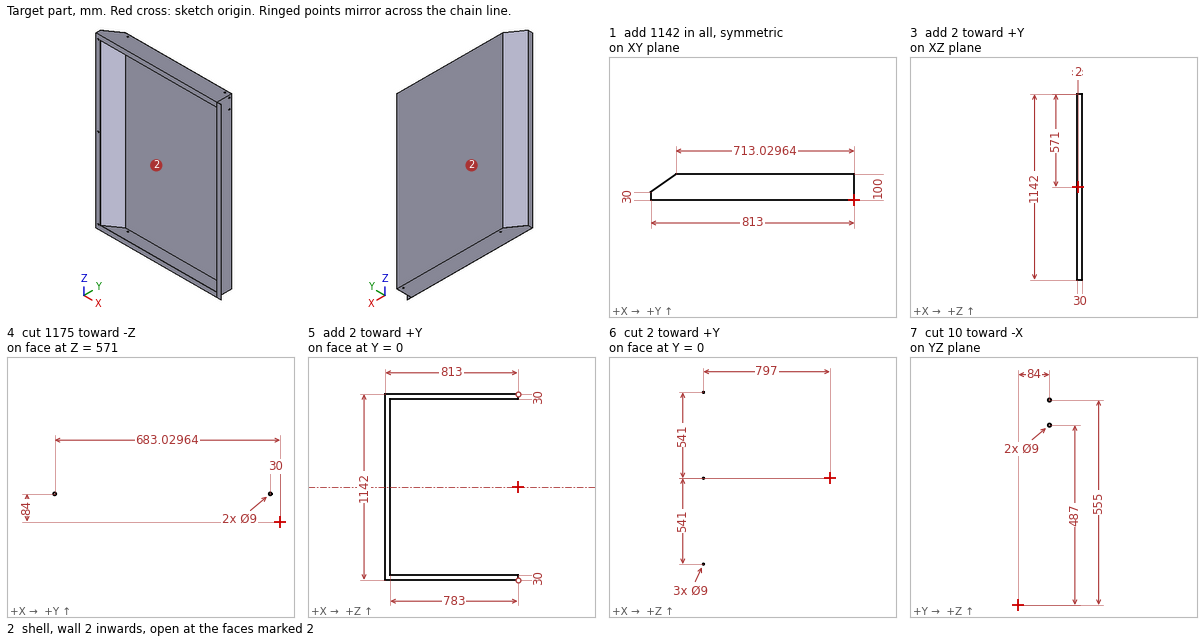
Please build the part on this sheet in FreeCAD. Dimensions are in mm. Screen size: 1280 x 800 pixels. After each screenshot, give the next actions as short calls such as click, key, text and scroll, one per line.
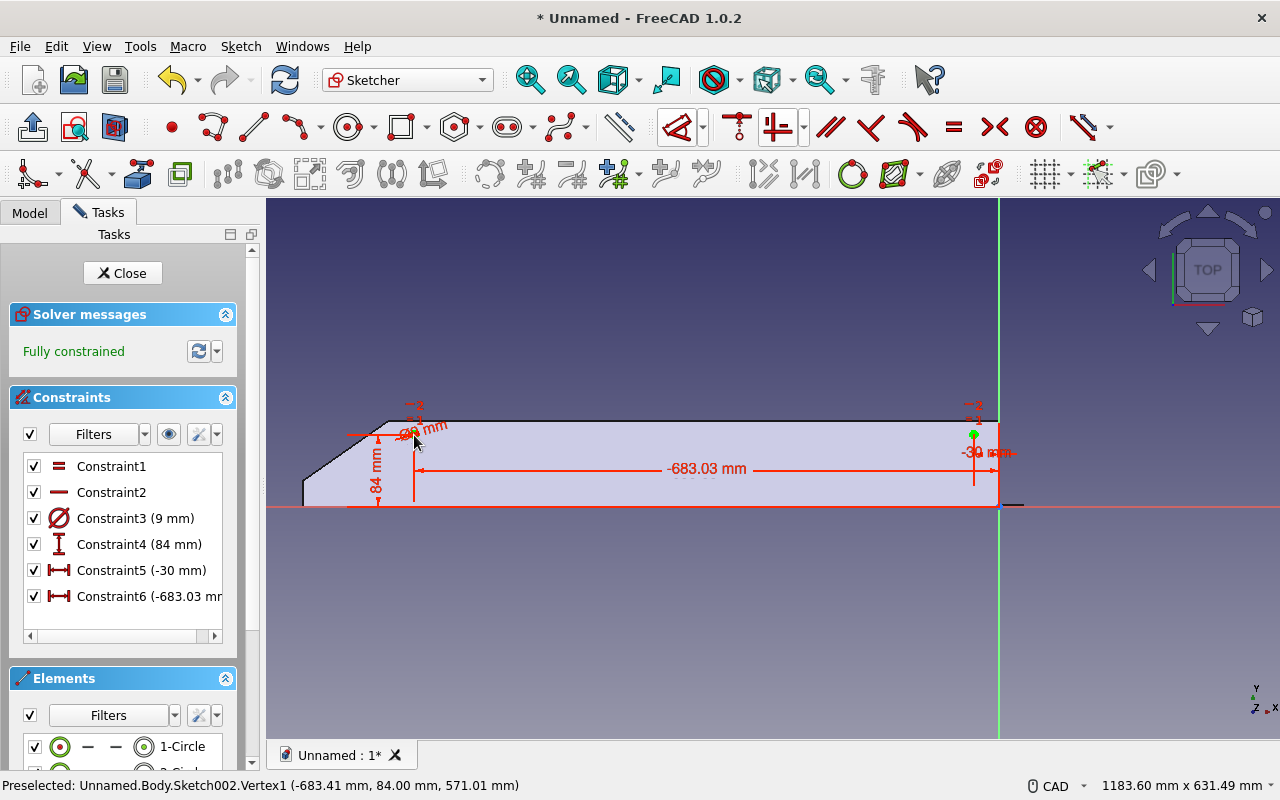
click(123, 273)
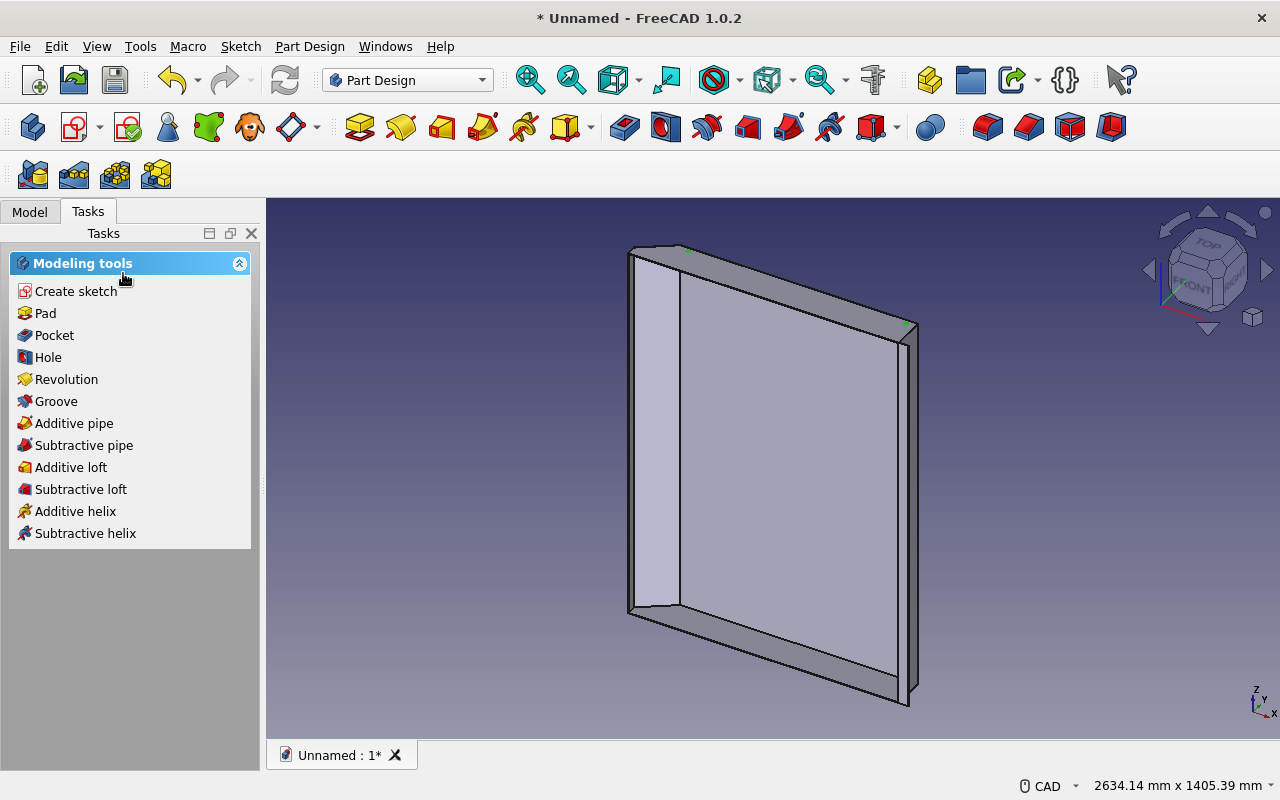
click(625, 128)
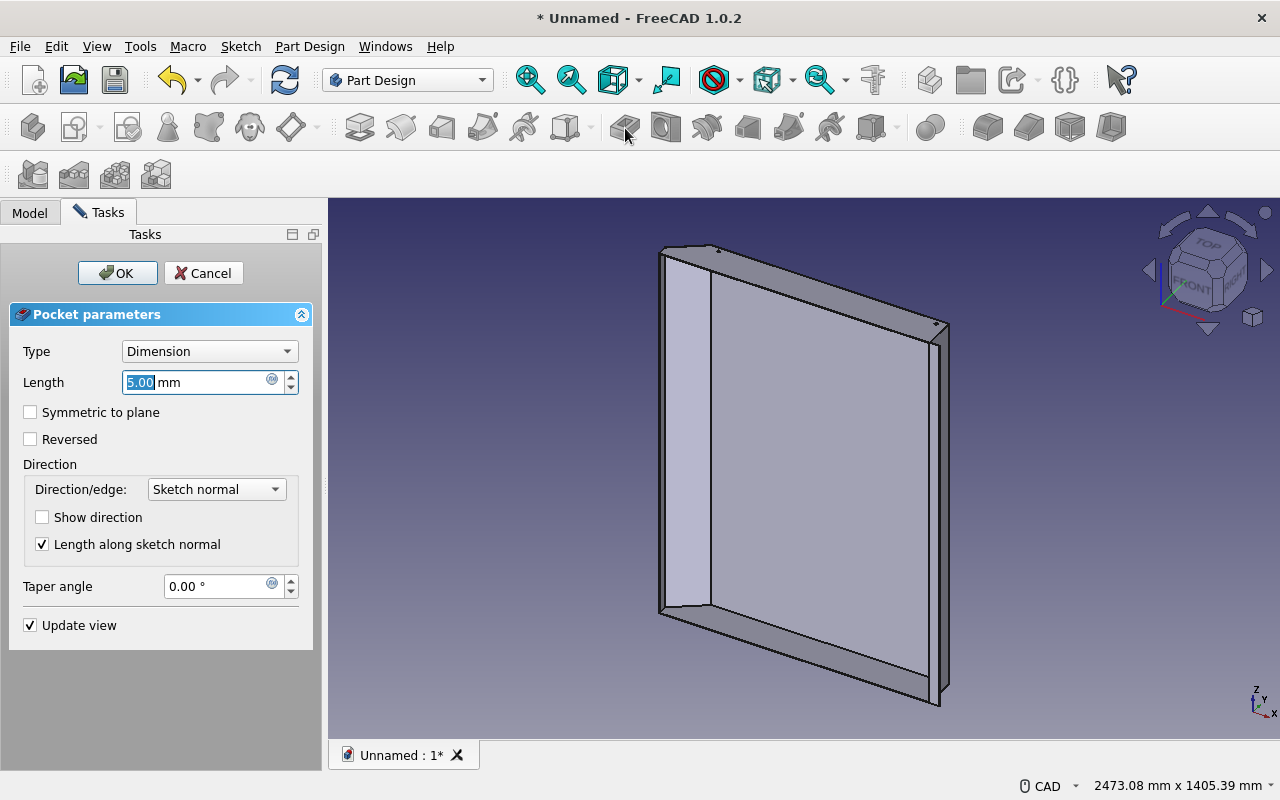
text(1175)
key(Tab)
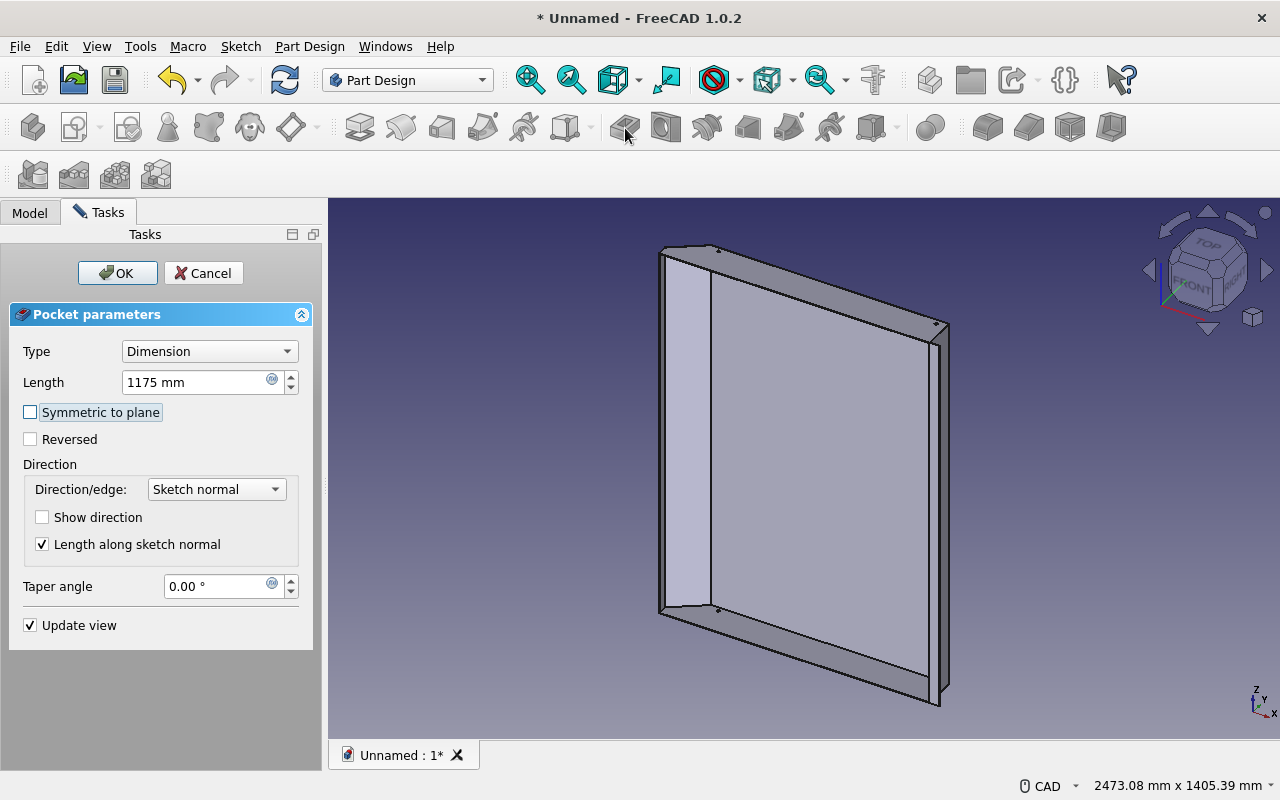
click(118, 273)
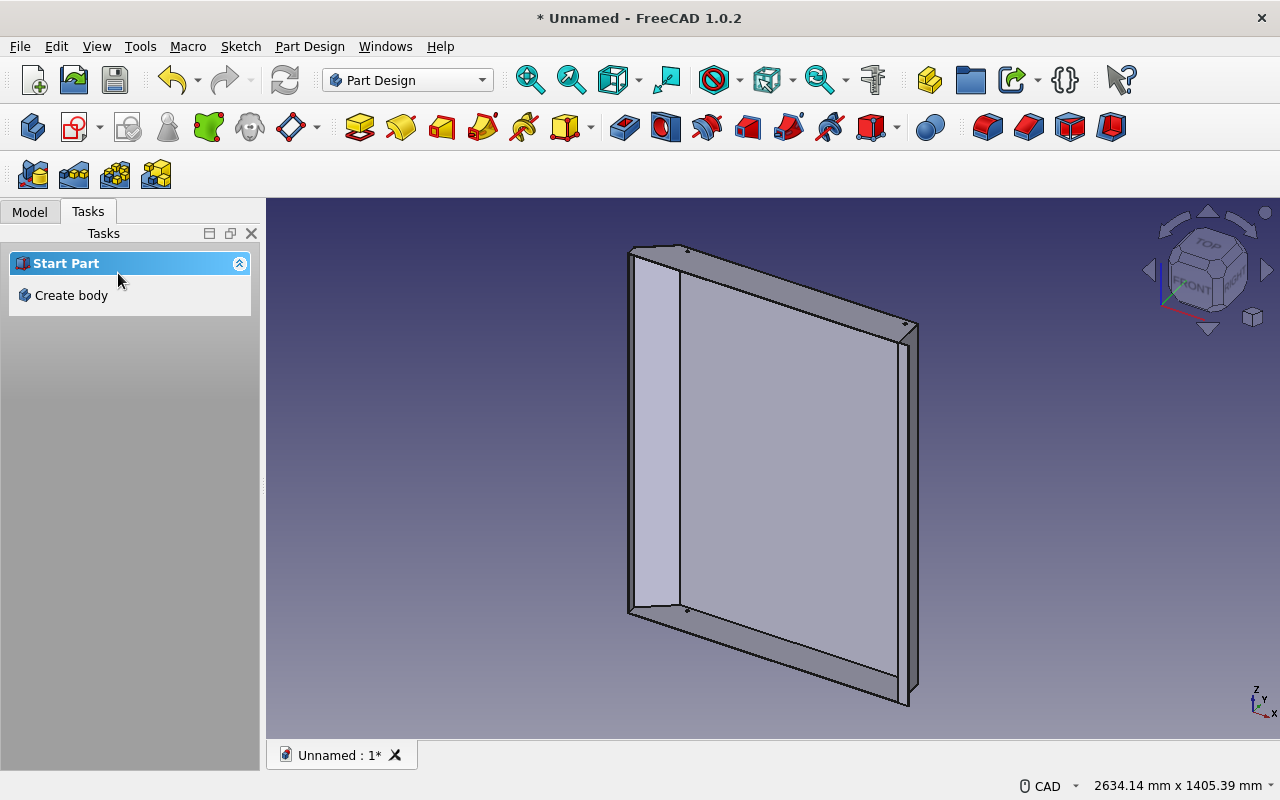
scroll(905, 584, up, 6)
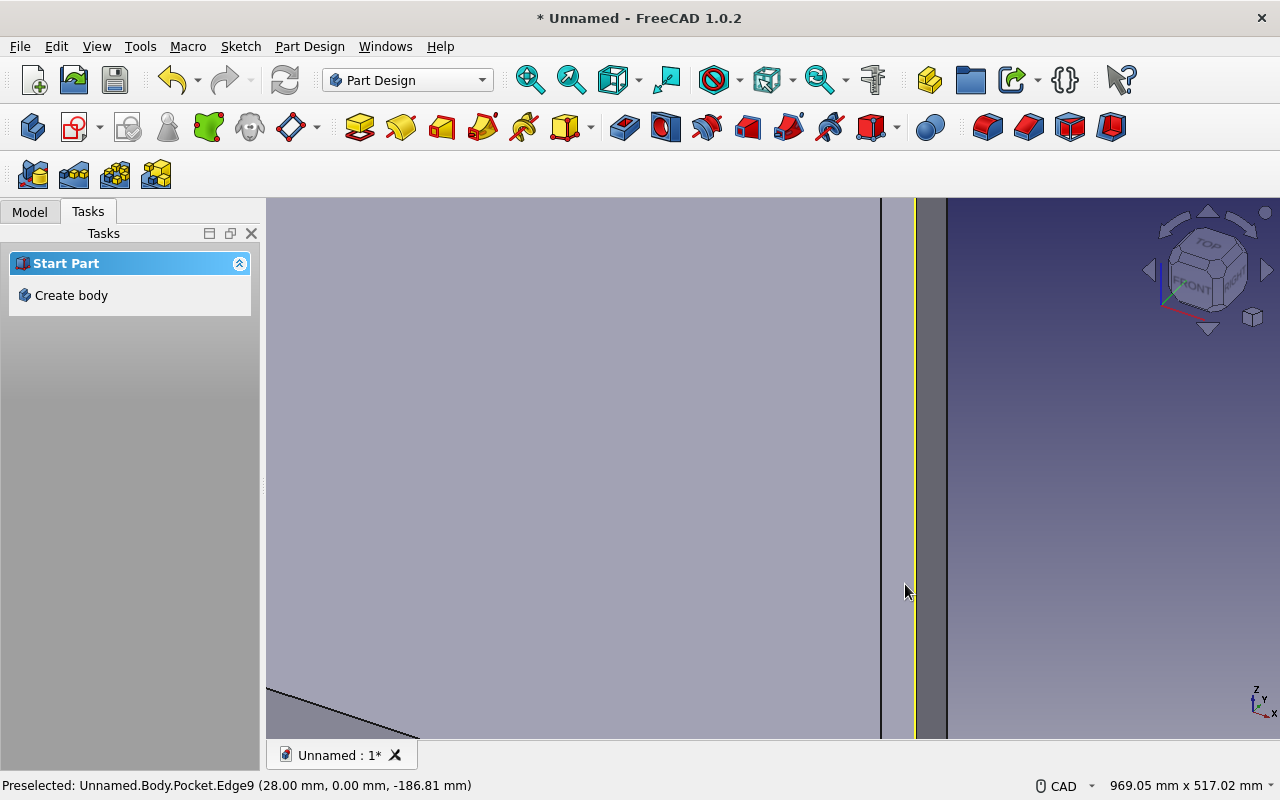
click(903, 584)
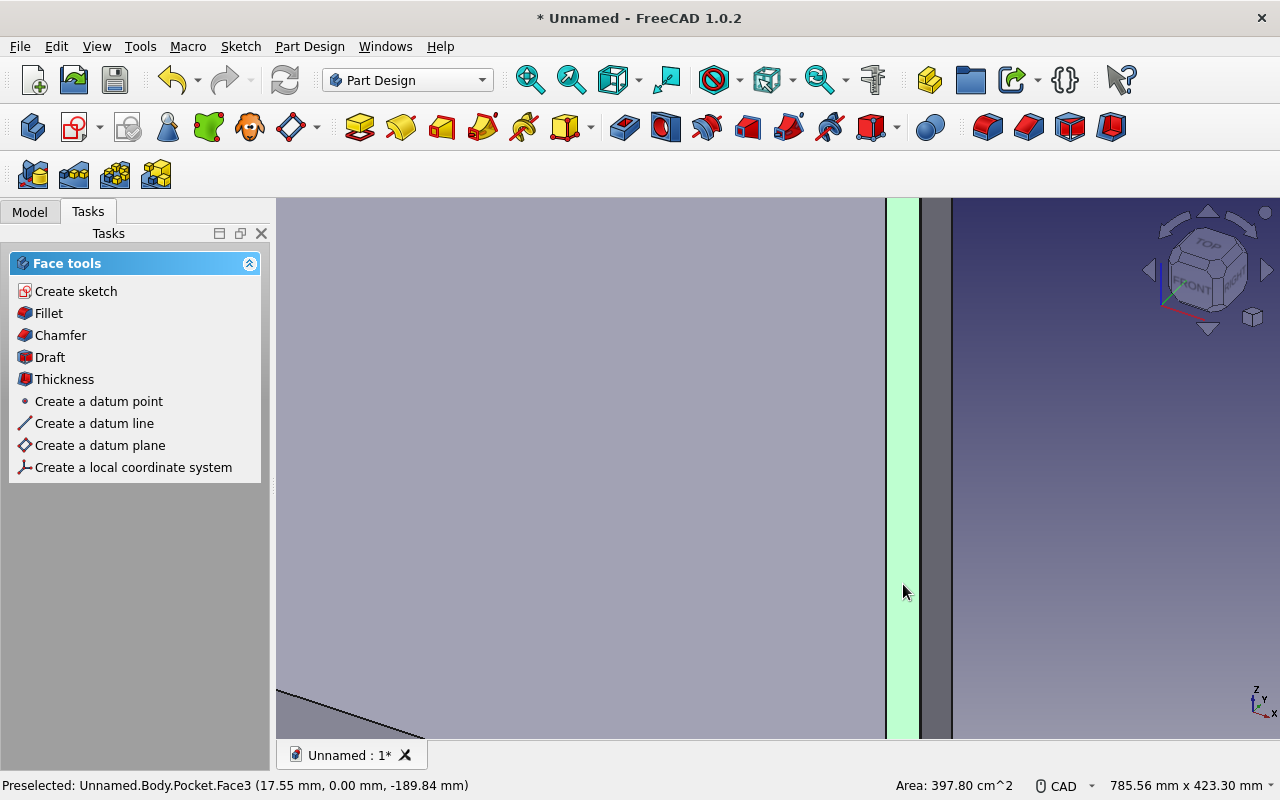
click(74, 128)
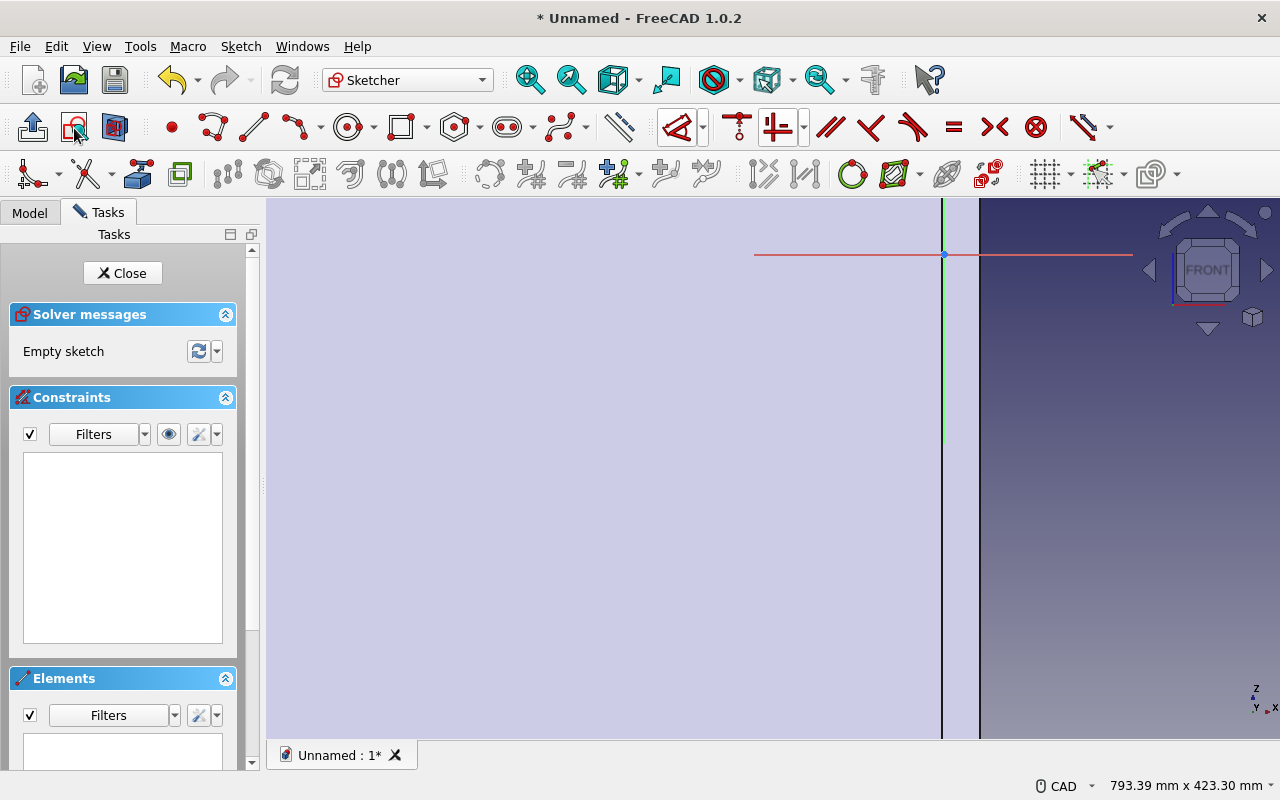
scroll(796, 539, down, 7)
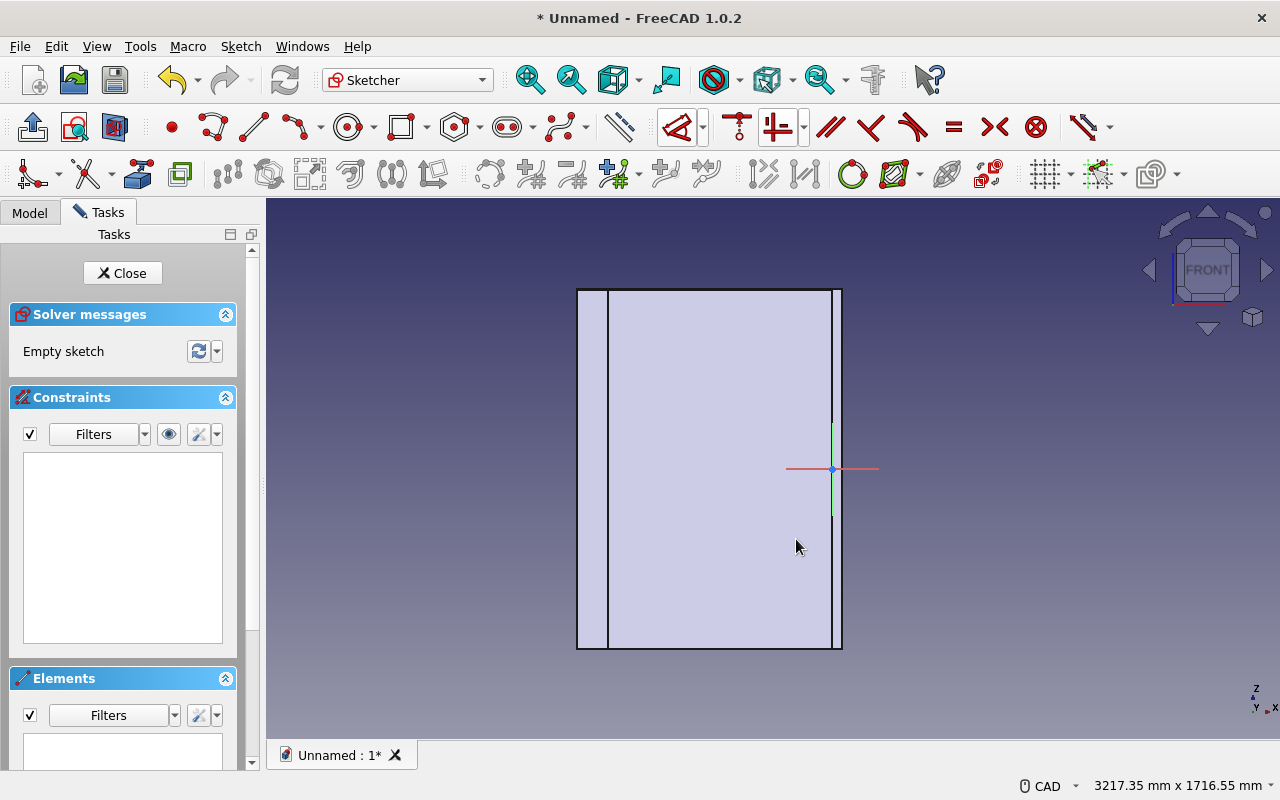
click(213, 128)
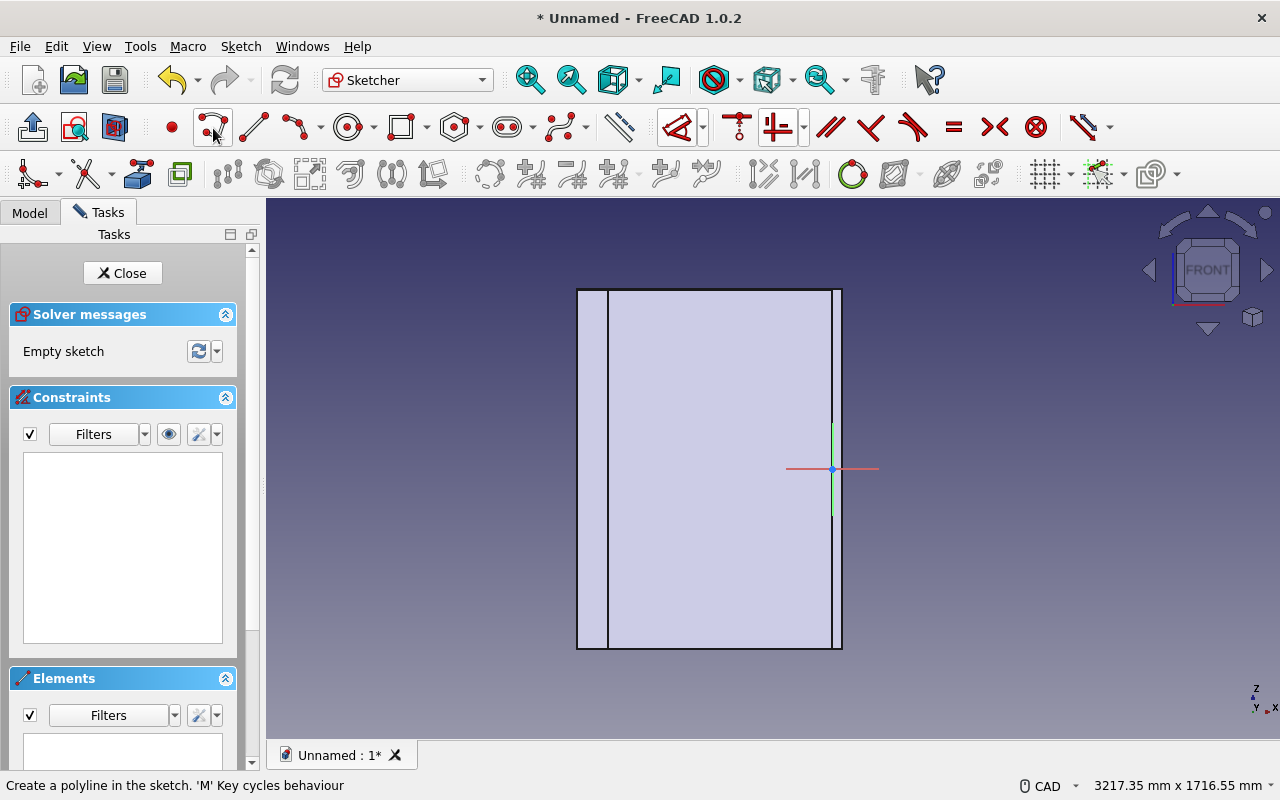
click(833, 299)